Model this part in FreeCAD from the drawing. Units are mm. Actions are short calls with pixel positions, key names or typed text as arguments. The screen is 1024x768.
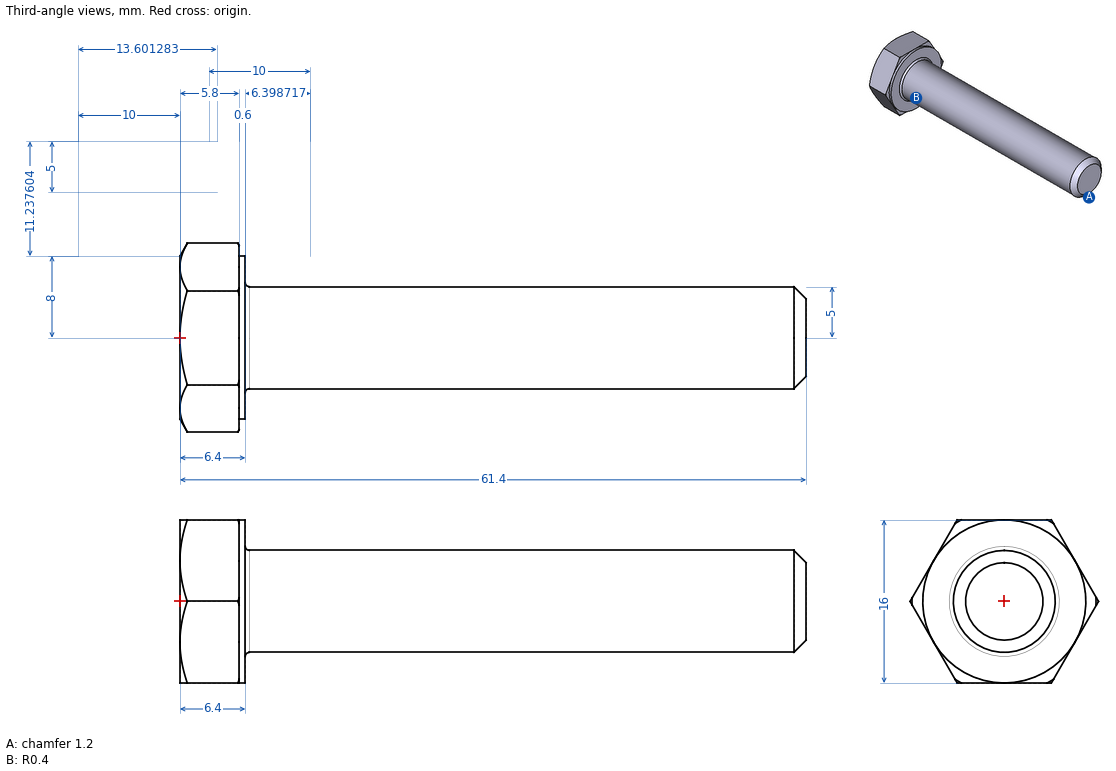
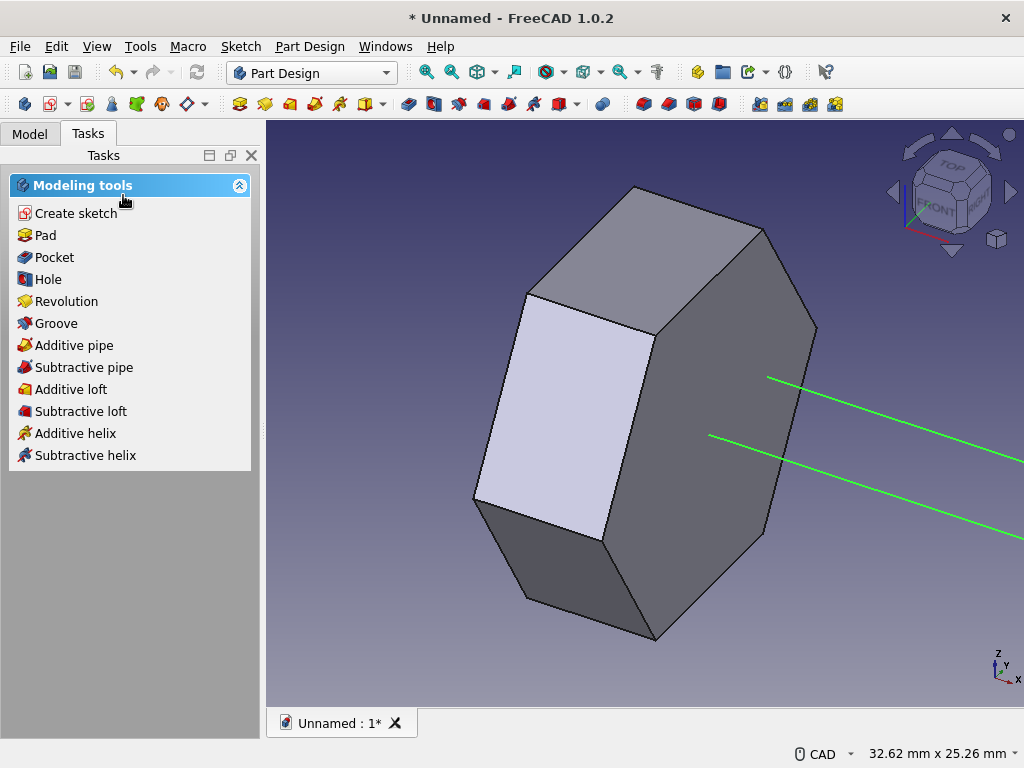
click(265, 104)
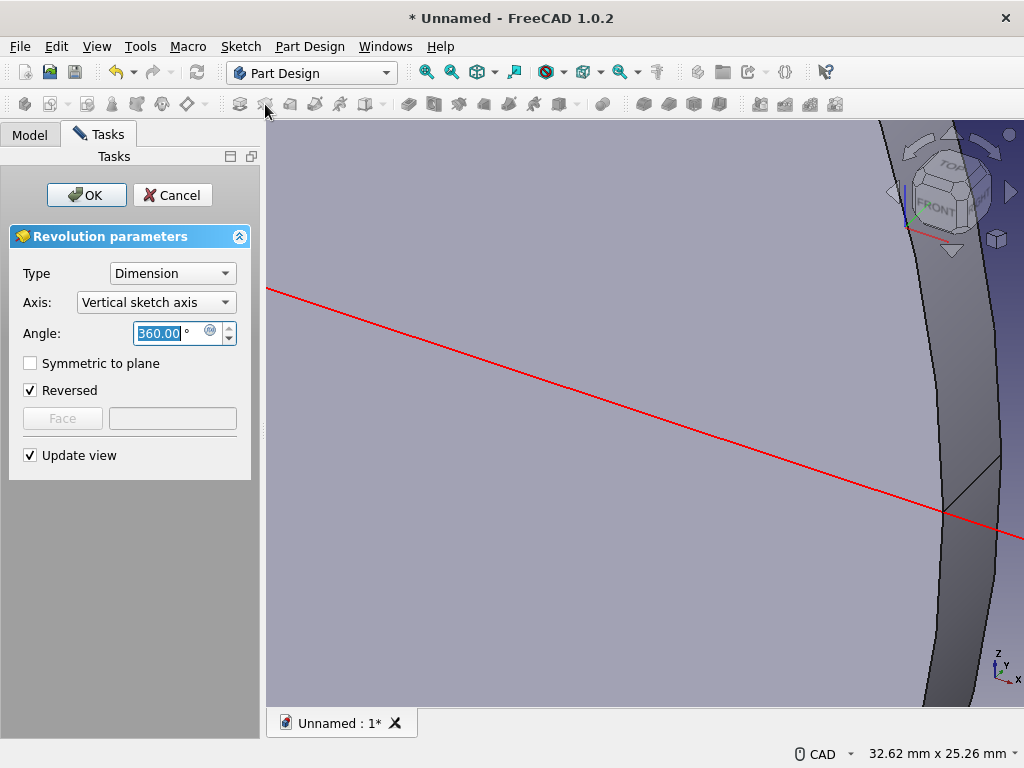
click(157, 302)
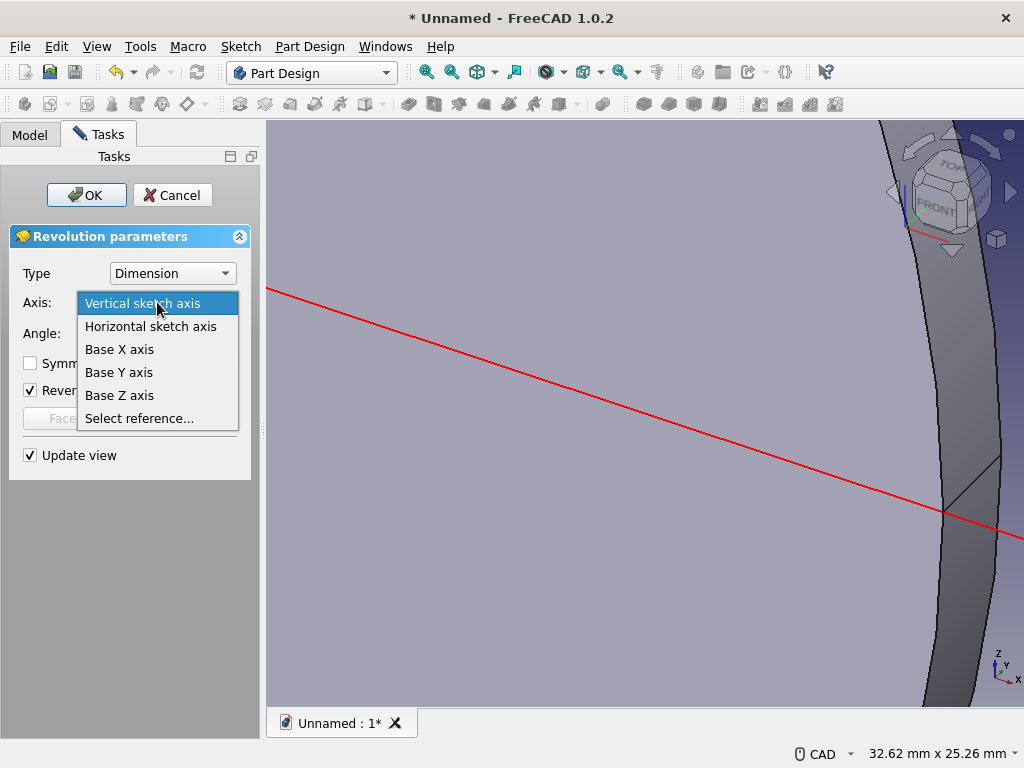
click(156, 326)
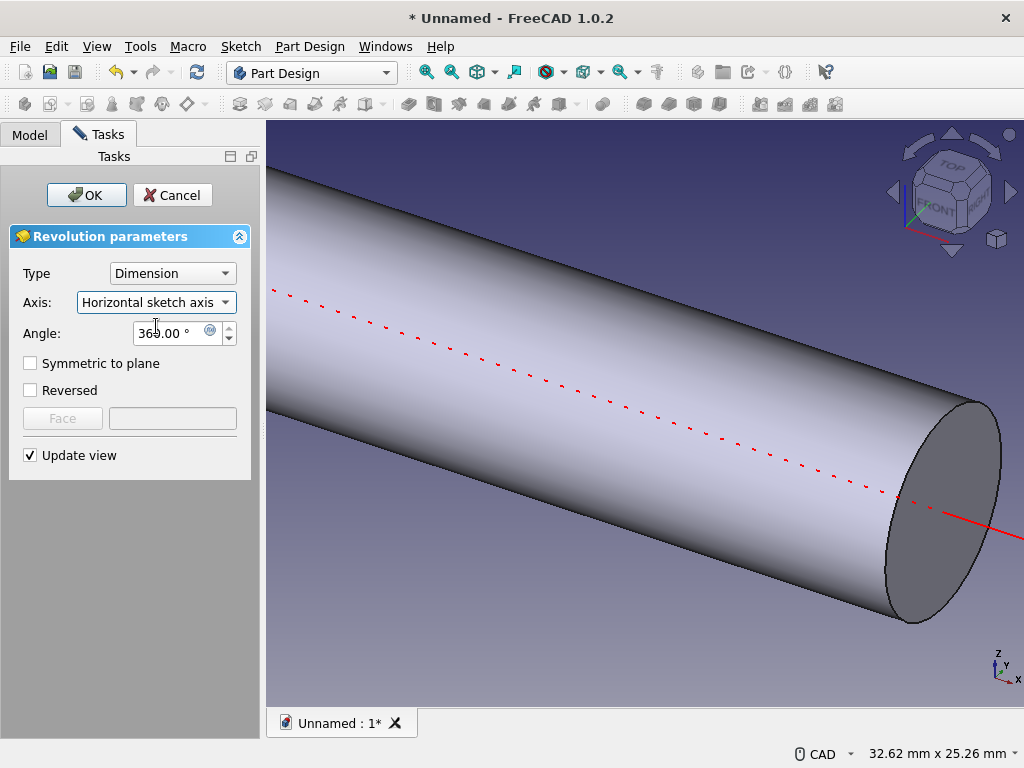
click(87, 195)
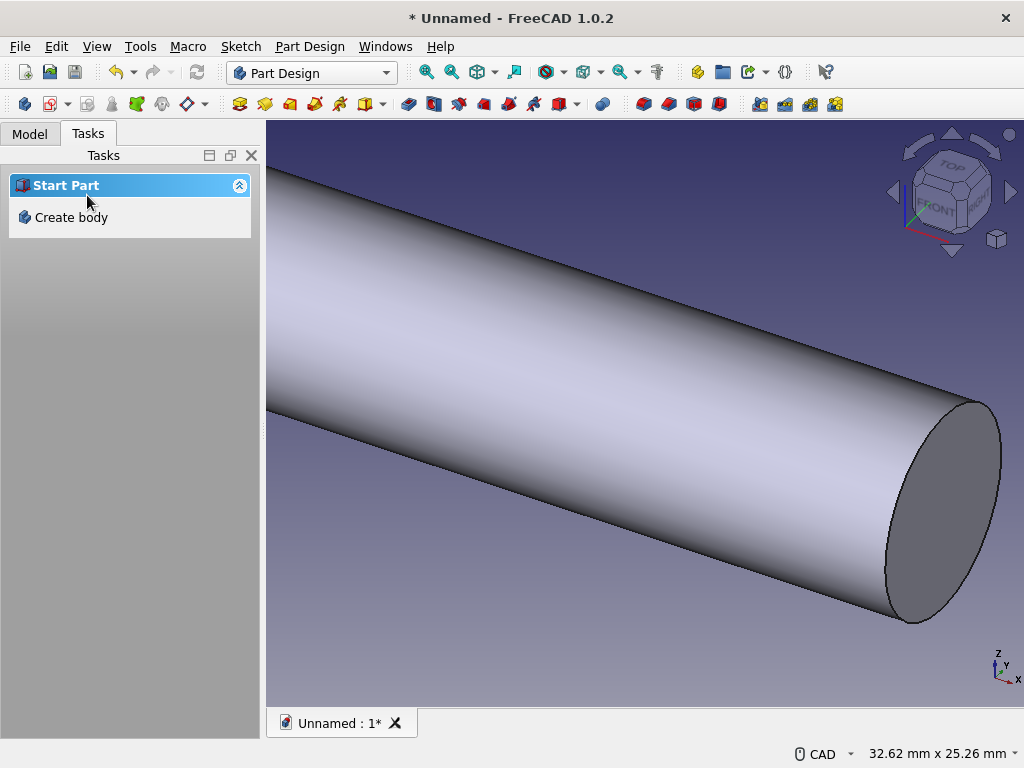
click(427, 72)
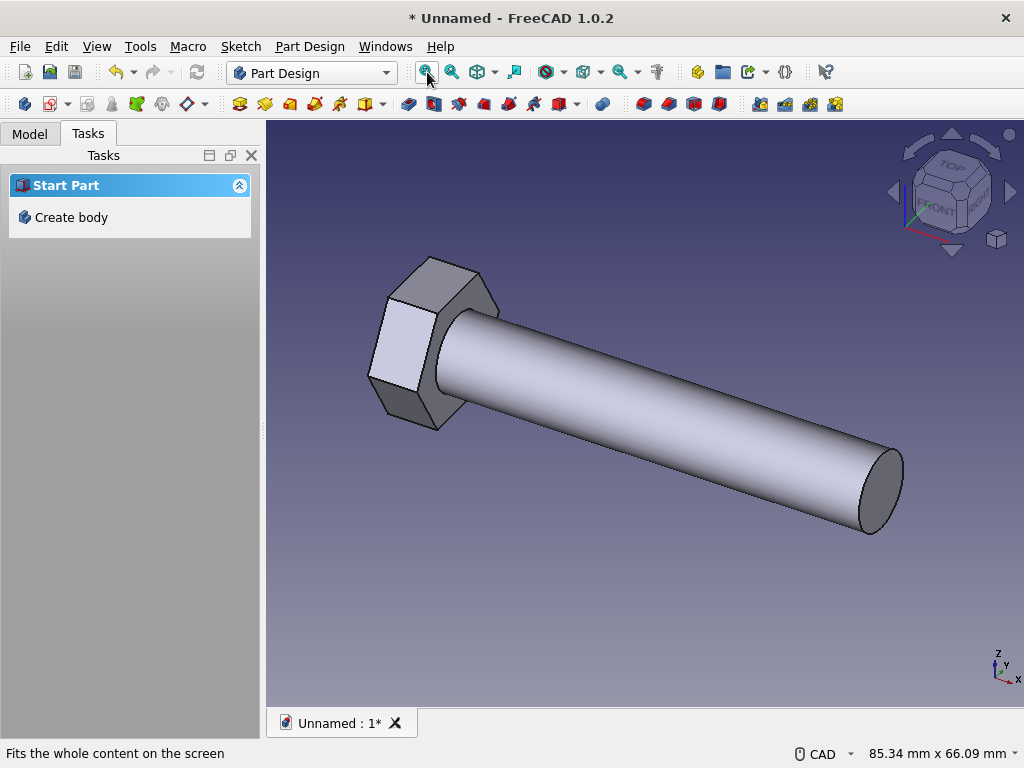
click(50, 104)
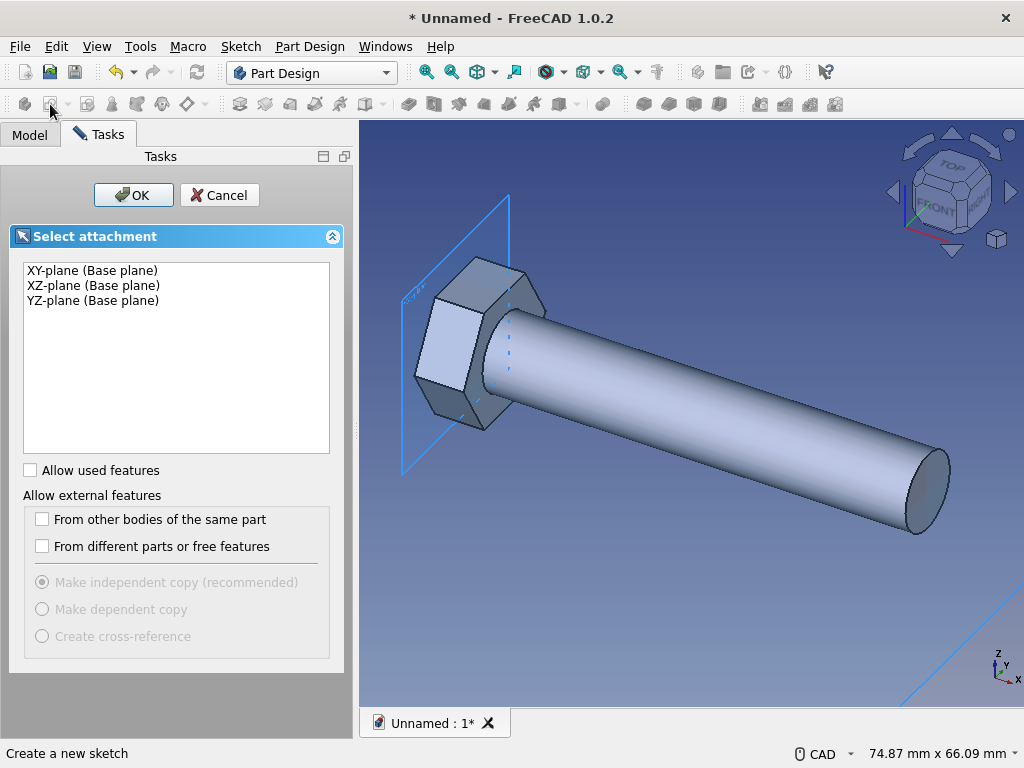
click(84, 270)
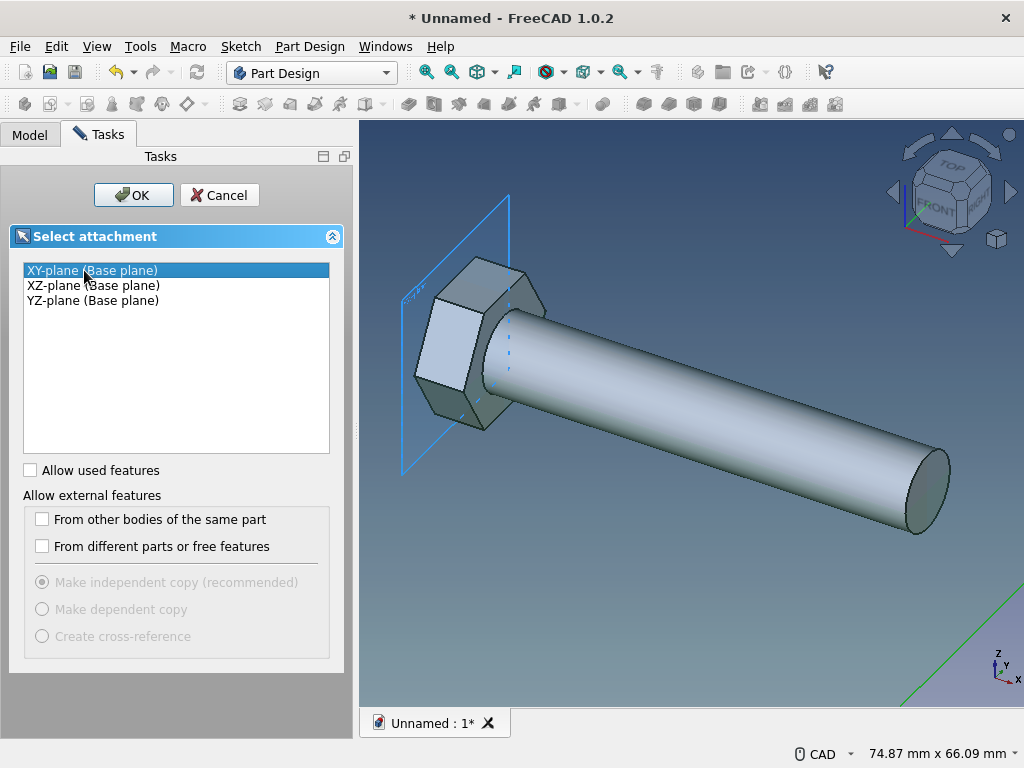
click(134, 195)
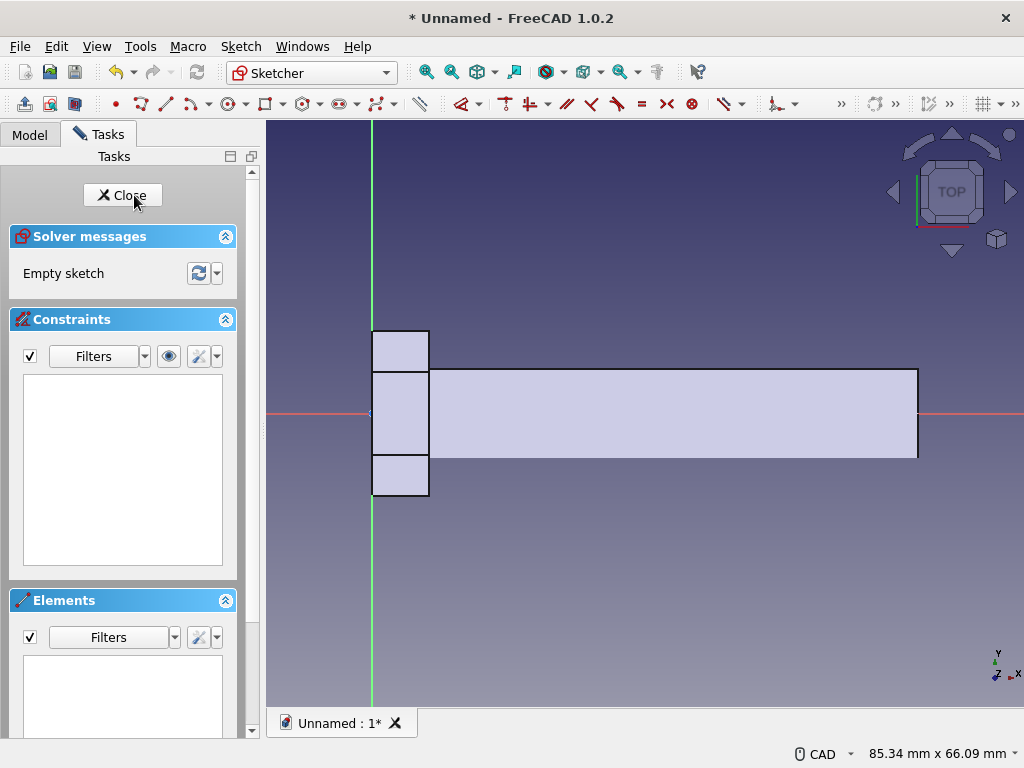
click(75, 104)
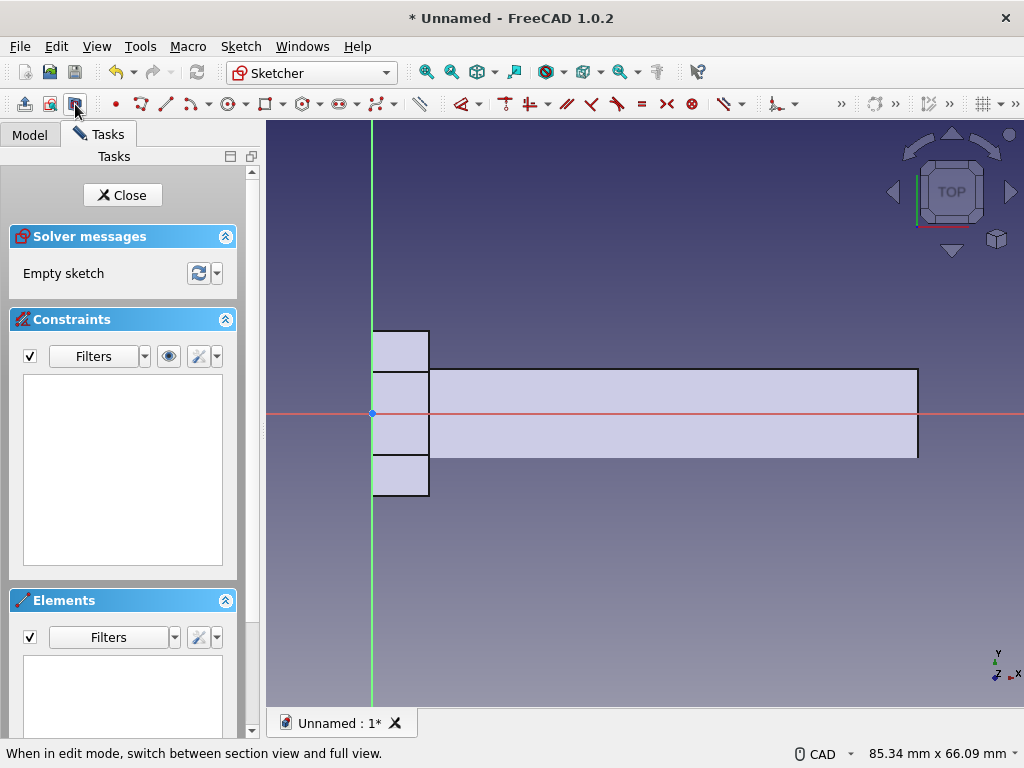
scroll(576, 414, down, 5)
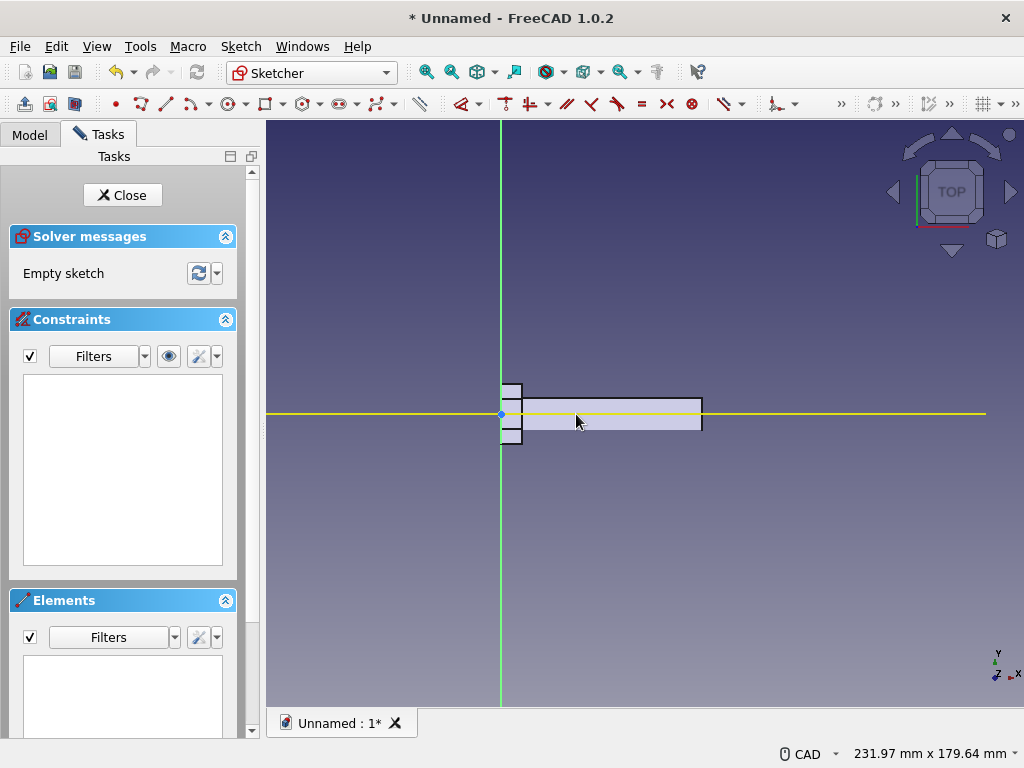
scroll(474, 377, up, 9)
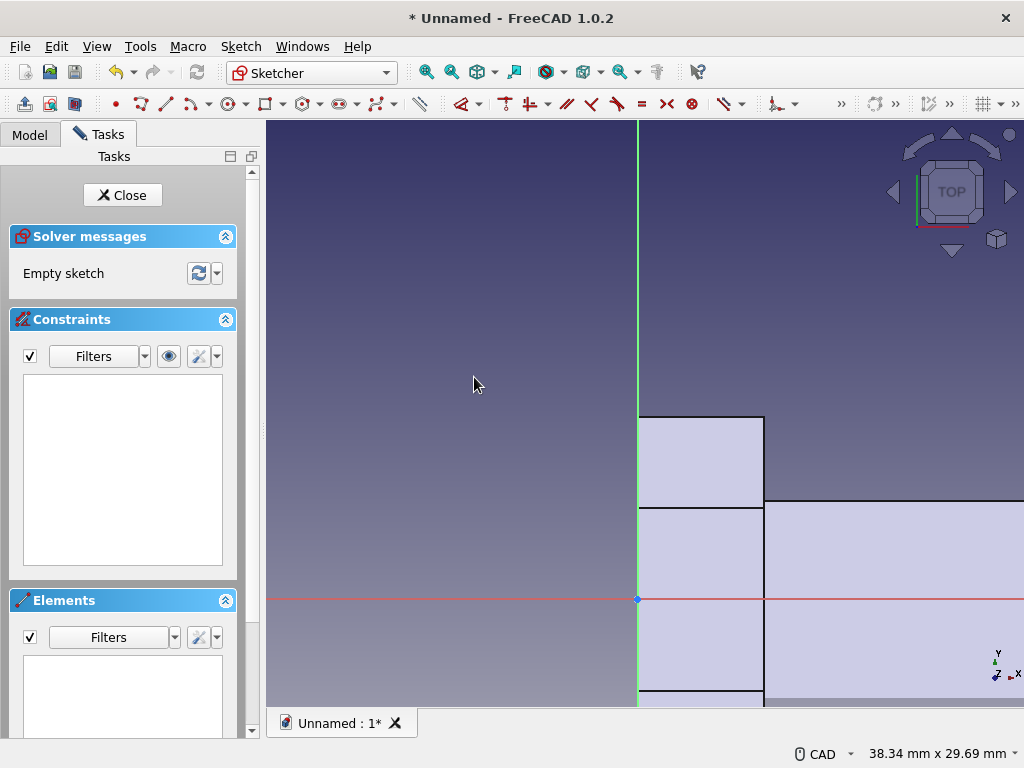
click(141, 104)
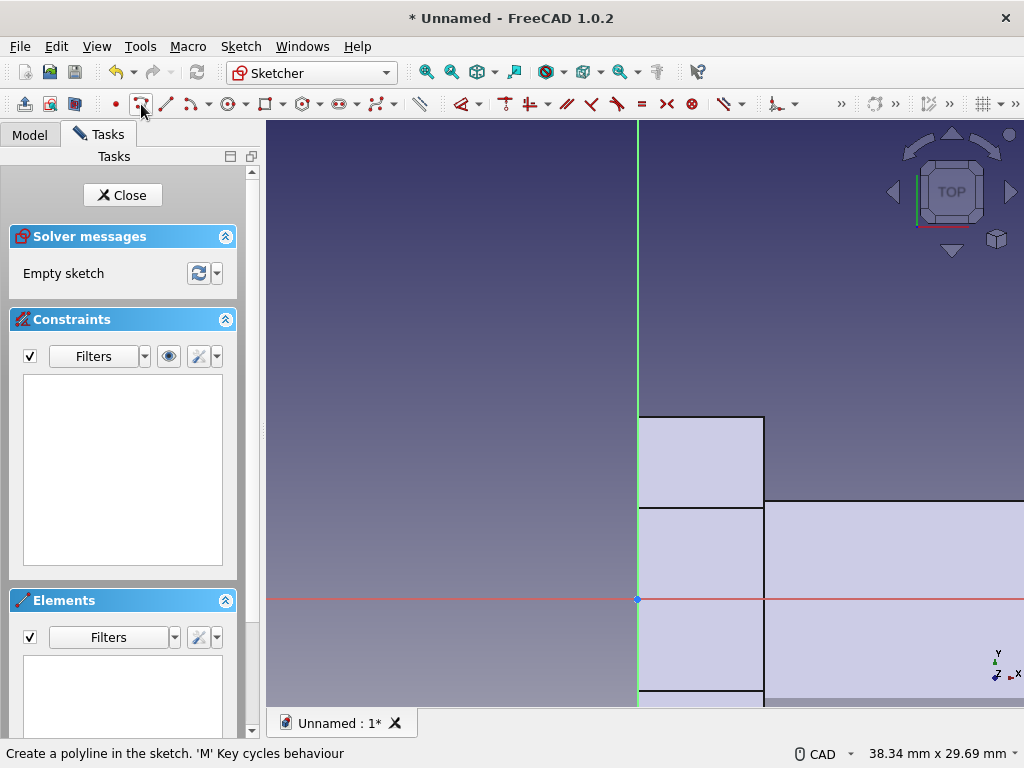
click(638, 441)
click(709, 318)
click(709, 219)
click(440, 219)
click(440, 441)
click(638, 442)
key(Escape)
key(Escape)